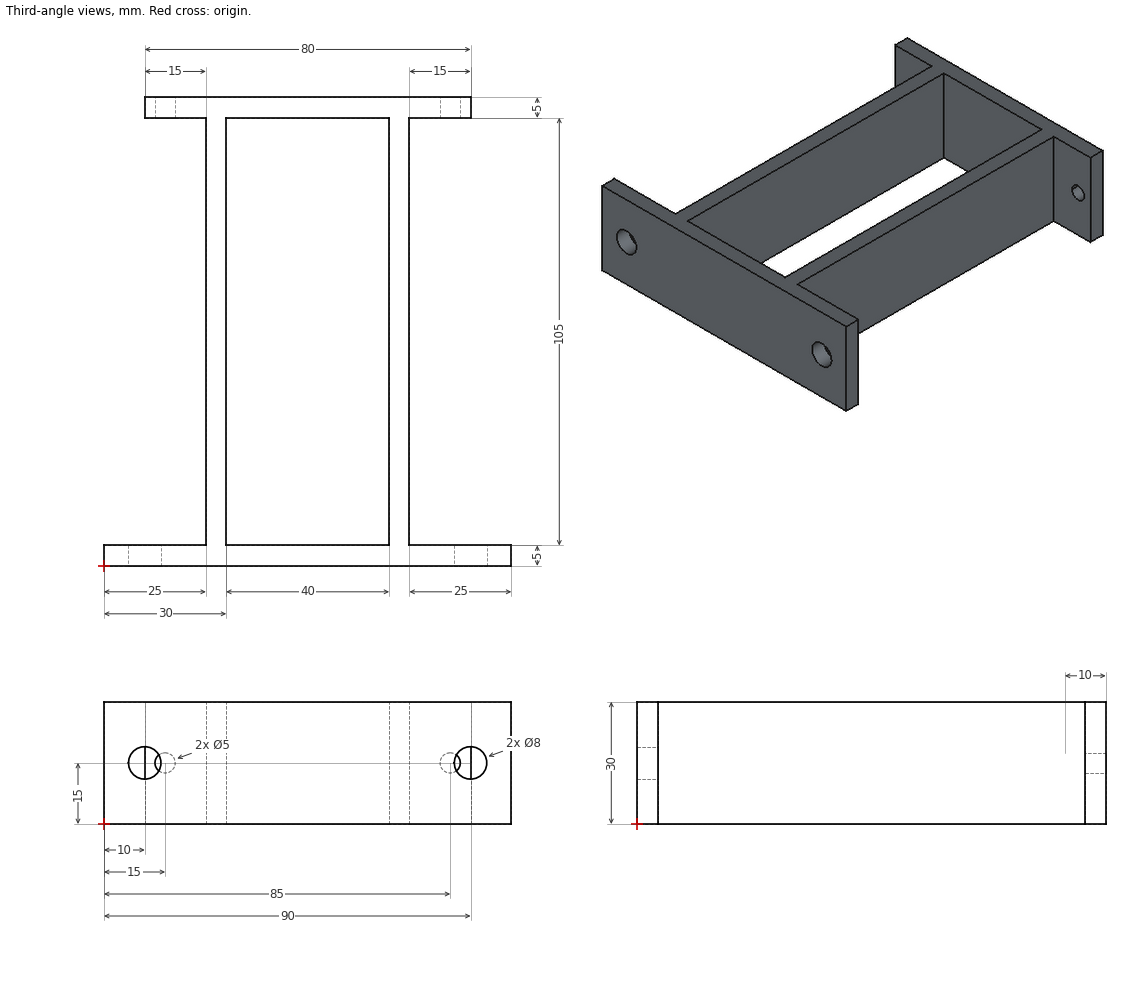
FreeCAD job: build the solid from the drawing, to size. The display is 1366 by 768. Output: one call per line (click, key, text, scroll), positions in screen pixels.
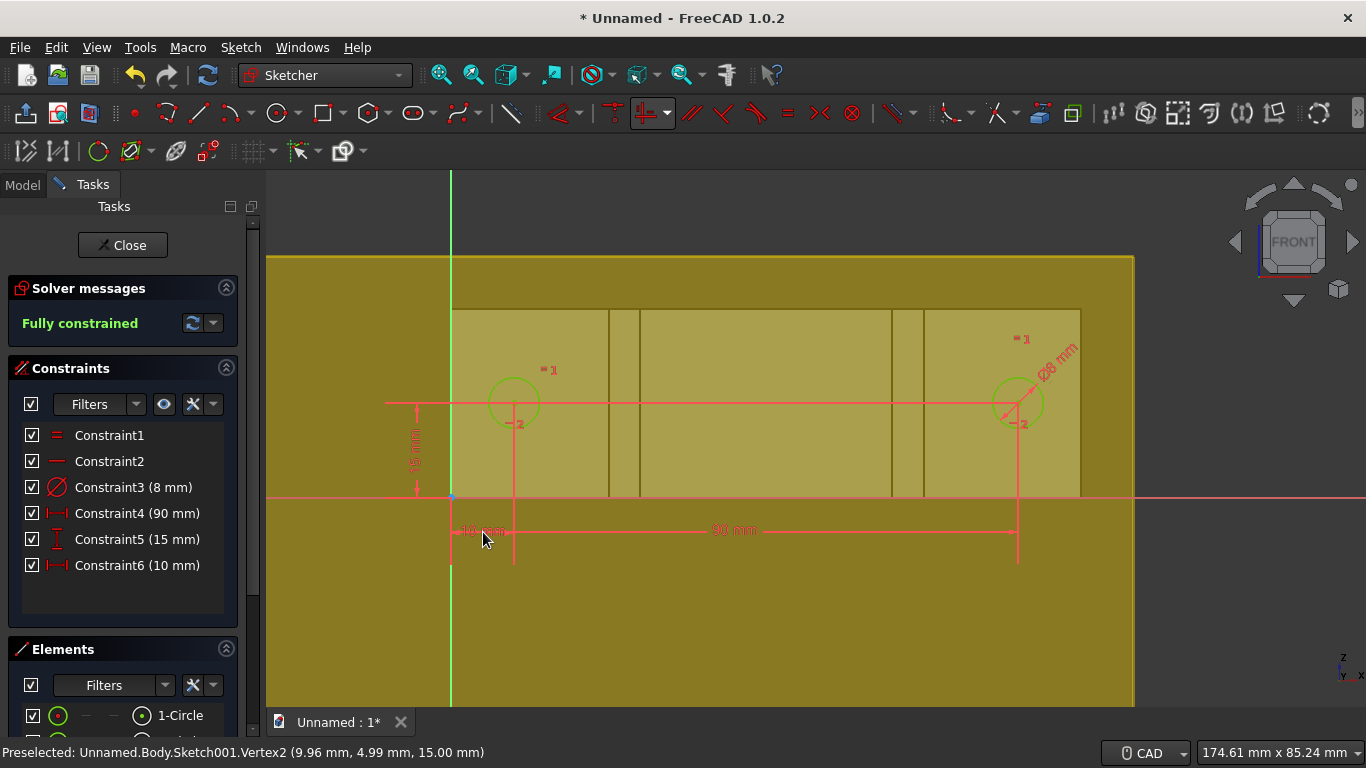
click(123, 245)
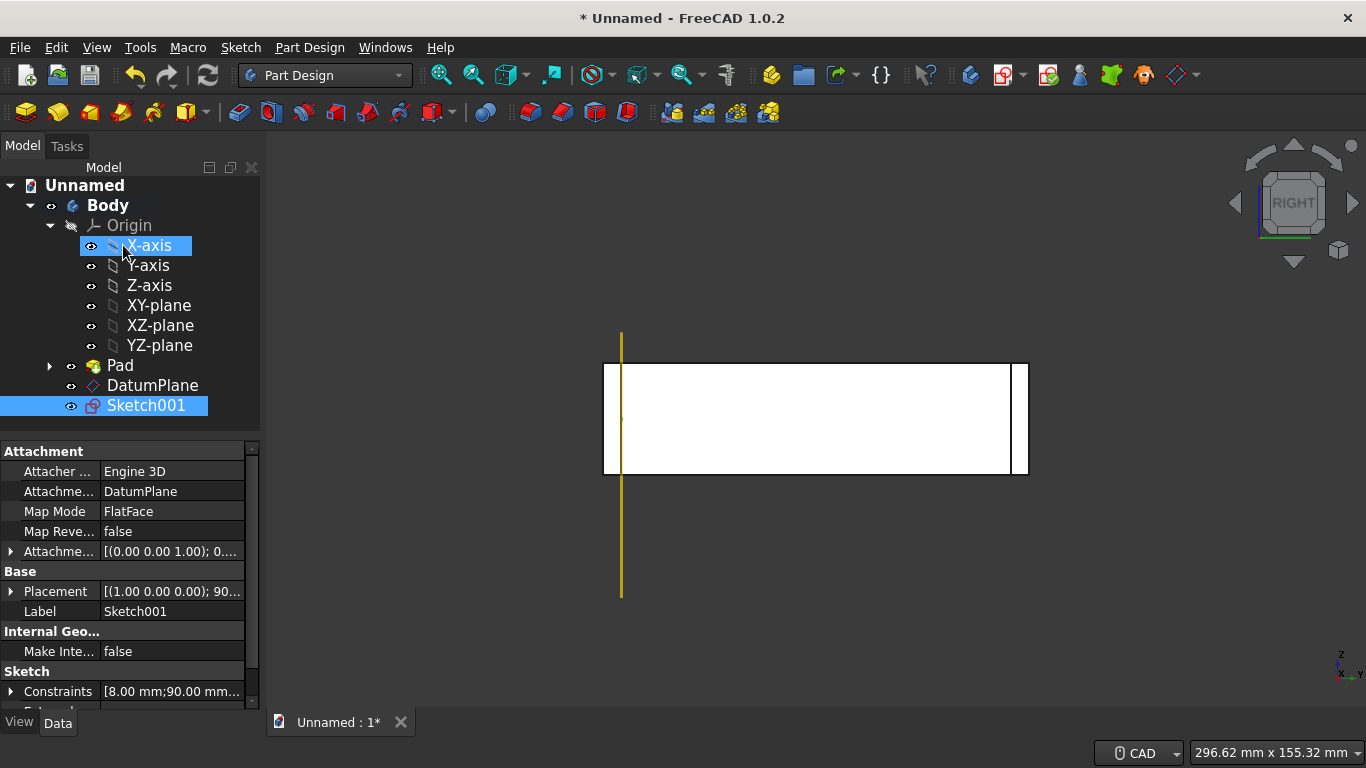
click(240, 112)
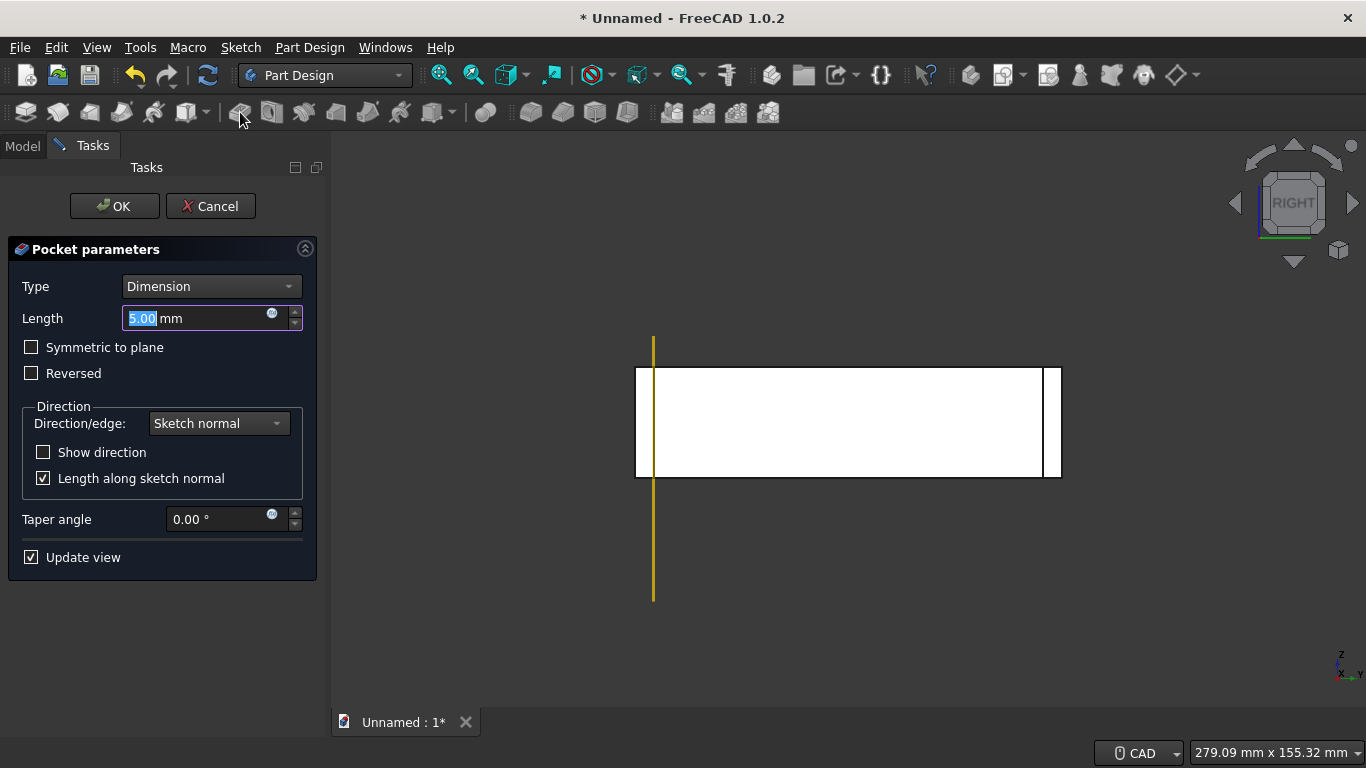
click(212, 286)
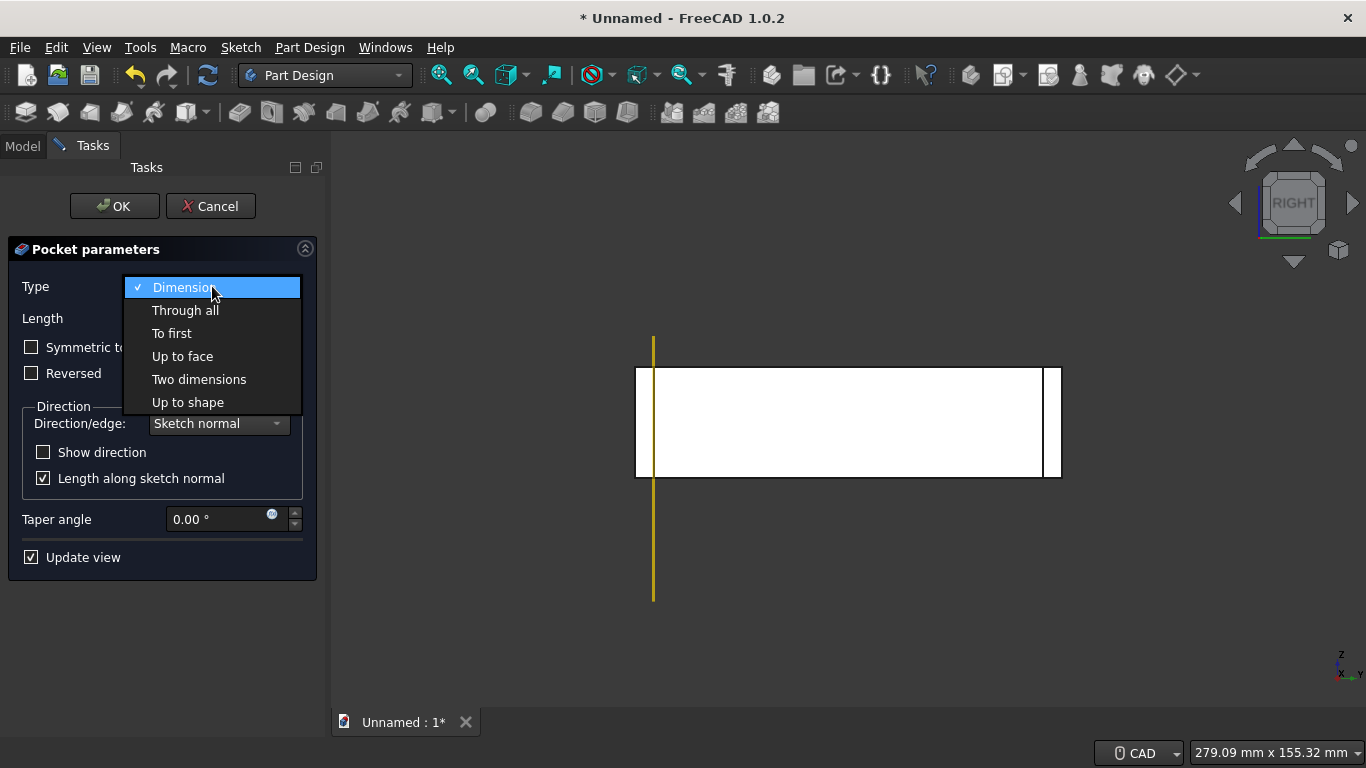
click(212, 310)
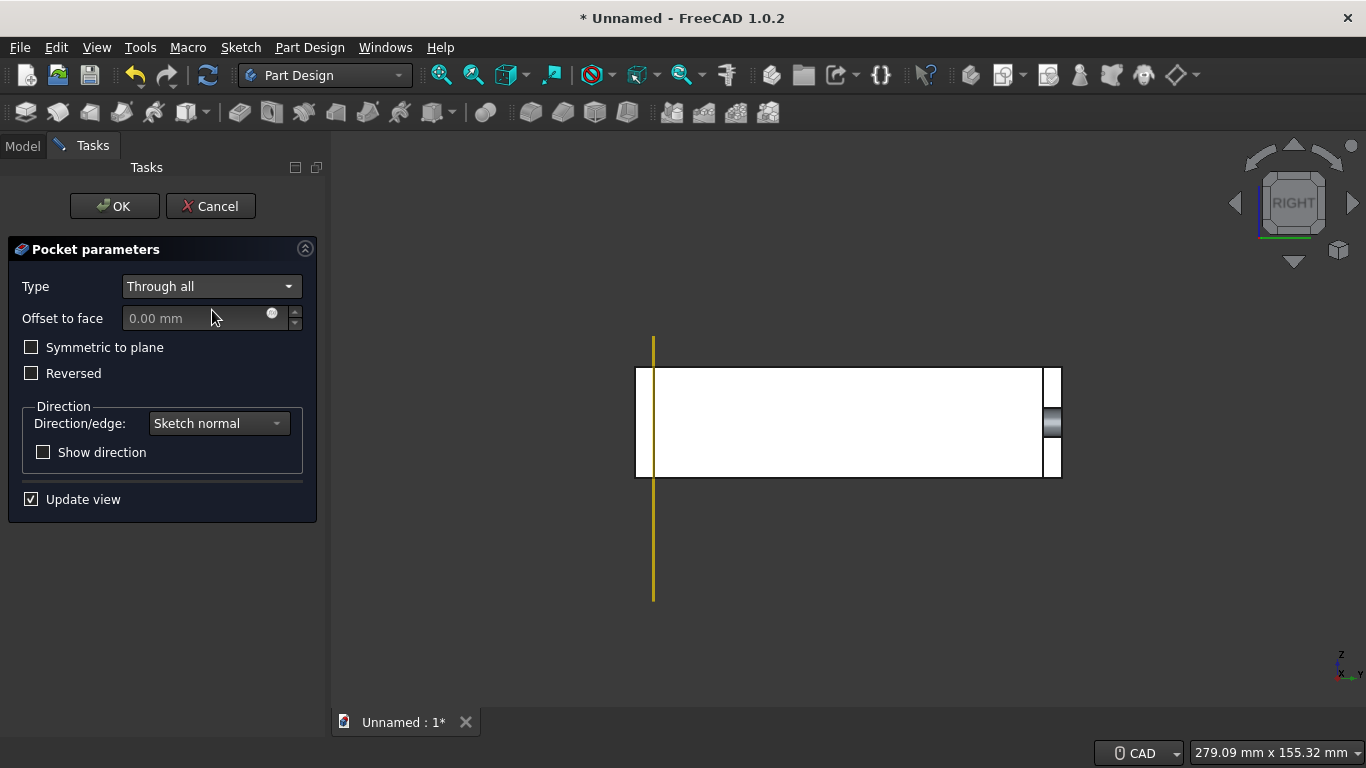
click(30, 373)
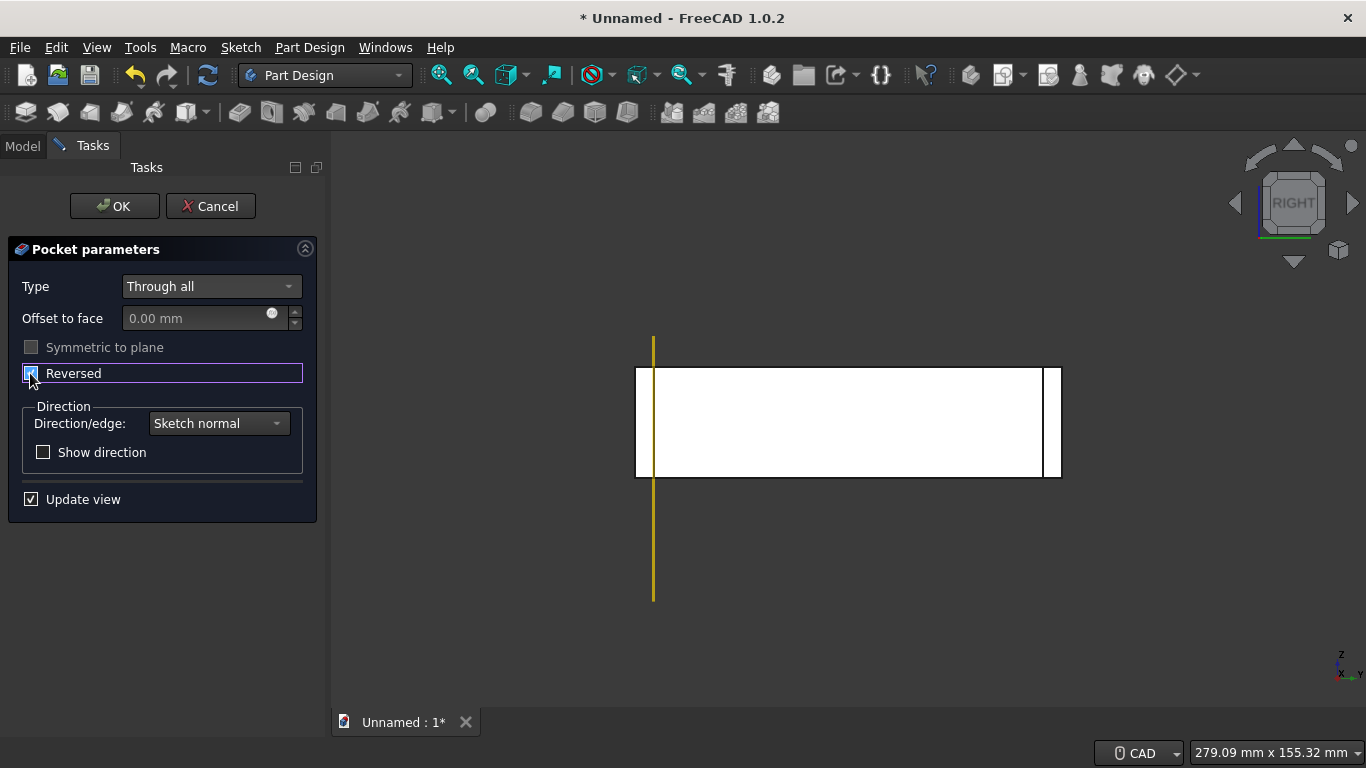
click(115, 206)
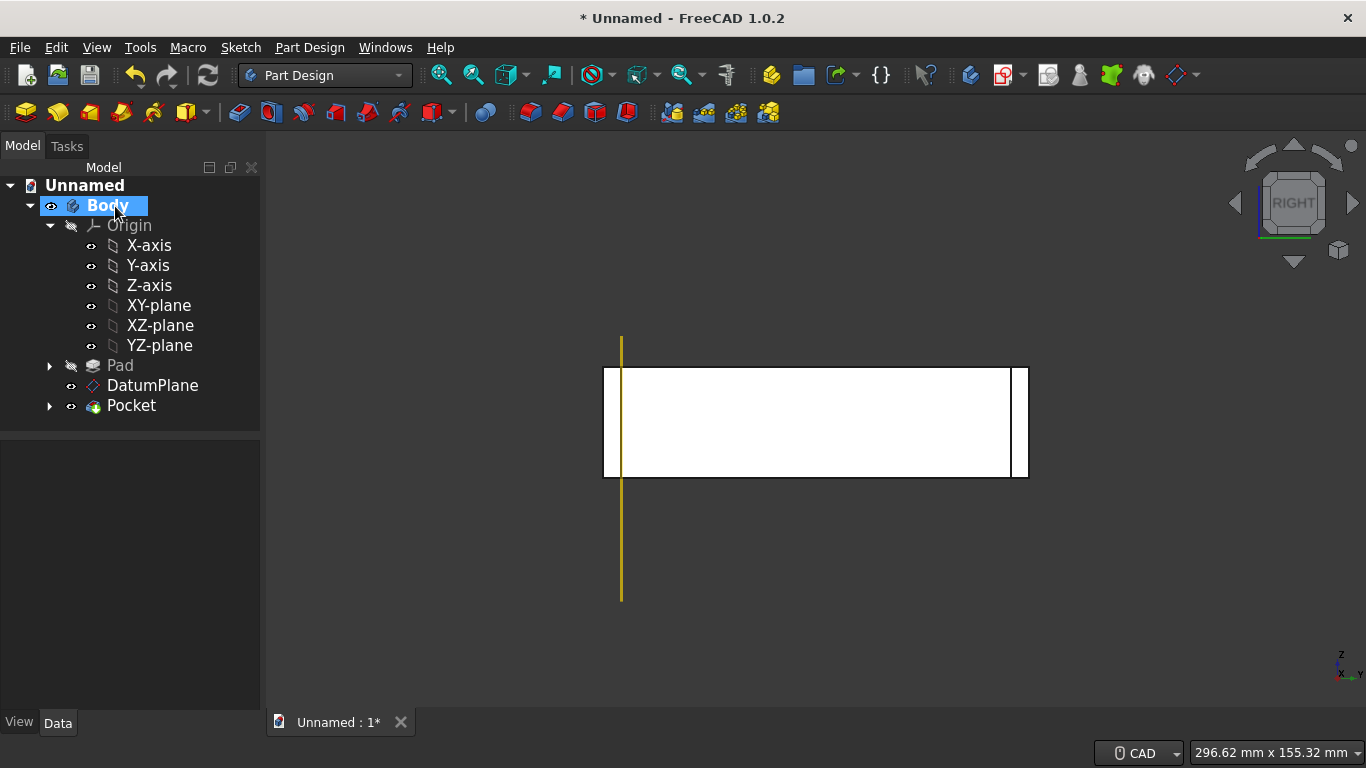
click(116, 386)
key(space)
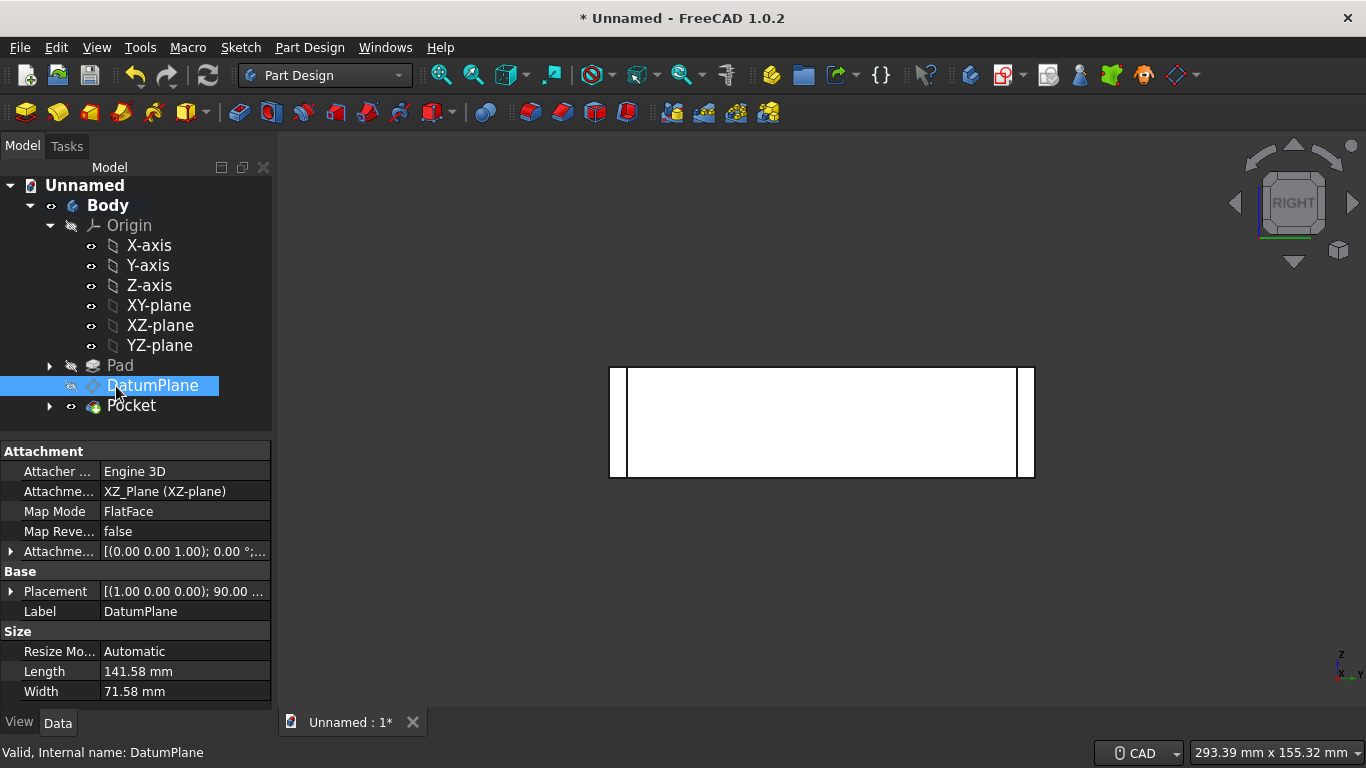
click(442, 76)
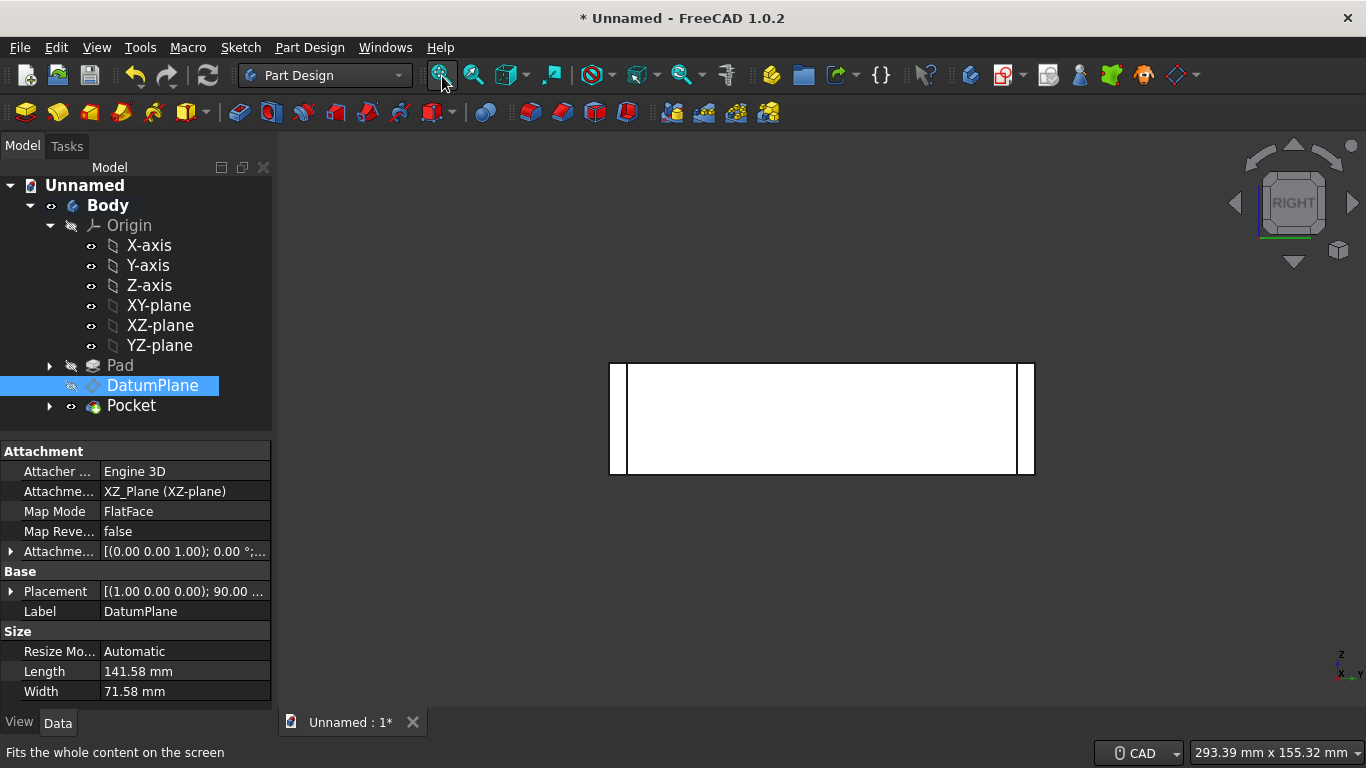
key(4)